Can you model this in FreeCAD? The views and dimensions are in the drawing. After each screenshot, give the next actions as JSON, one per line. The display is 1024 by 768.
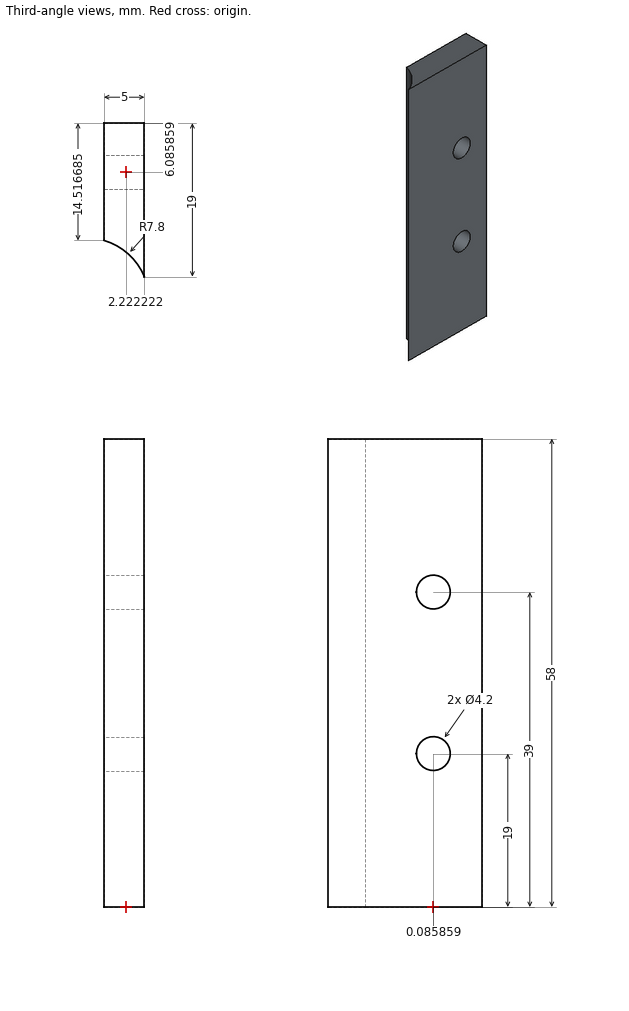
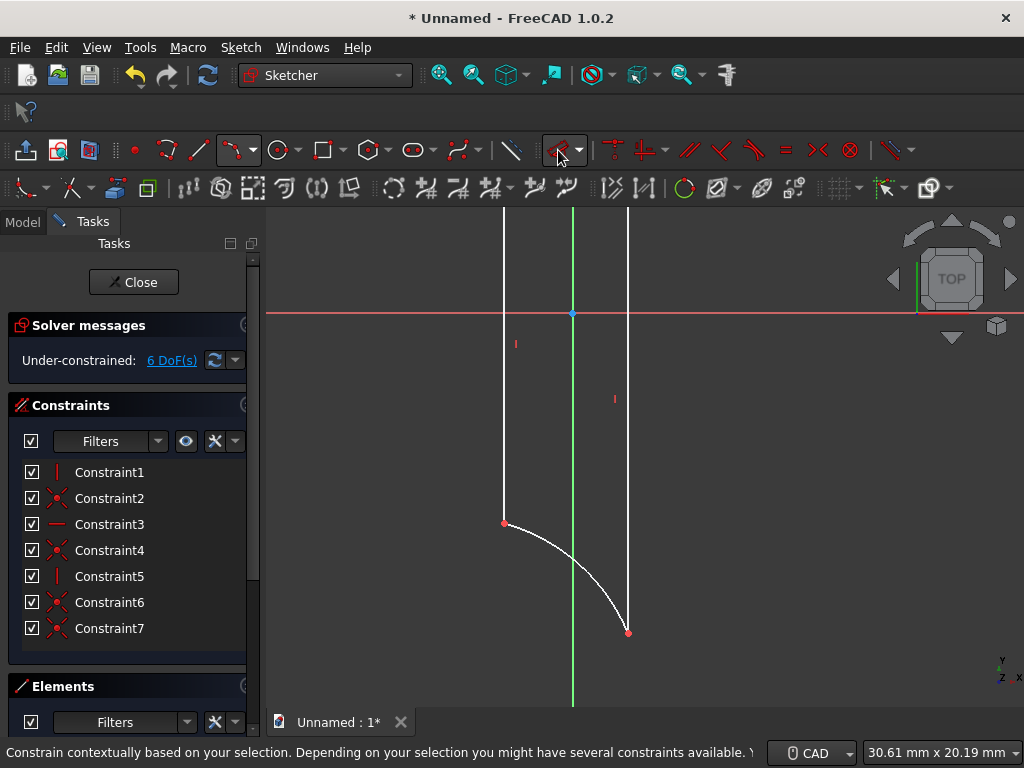
{"action": "left_click", "coordinate": [602, 589]}
{"action": "left_click", "coordinate": [671, 669]}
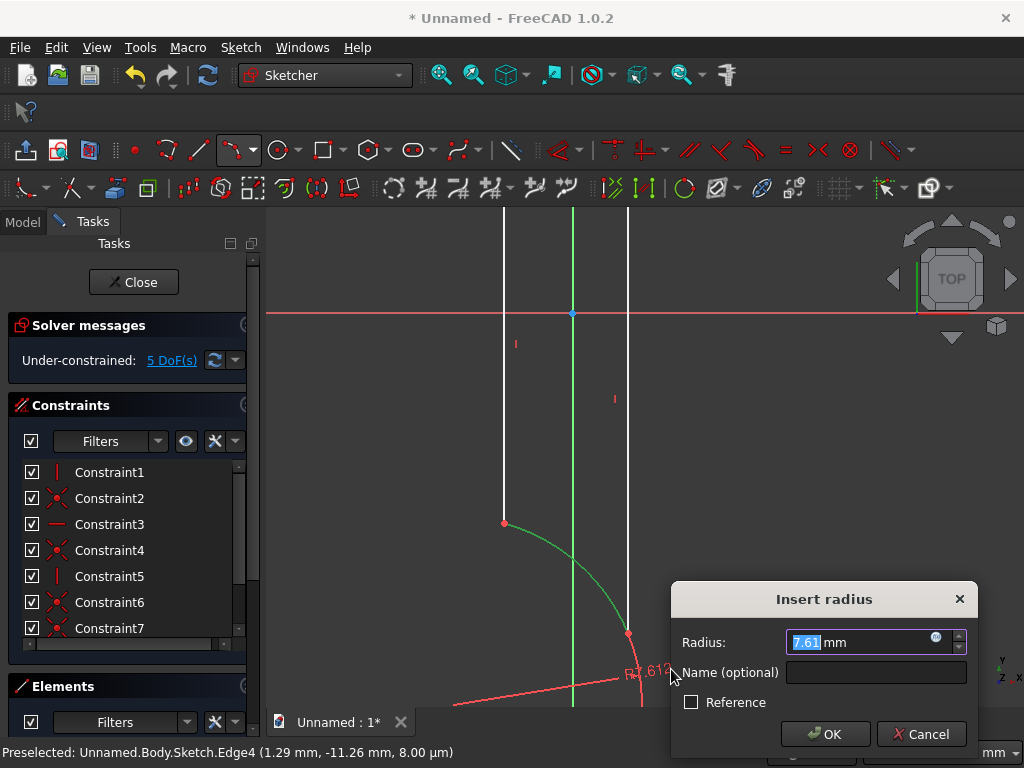
{"action": "type", "text": "7.8"}
{"action": "key", "text": "Return"}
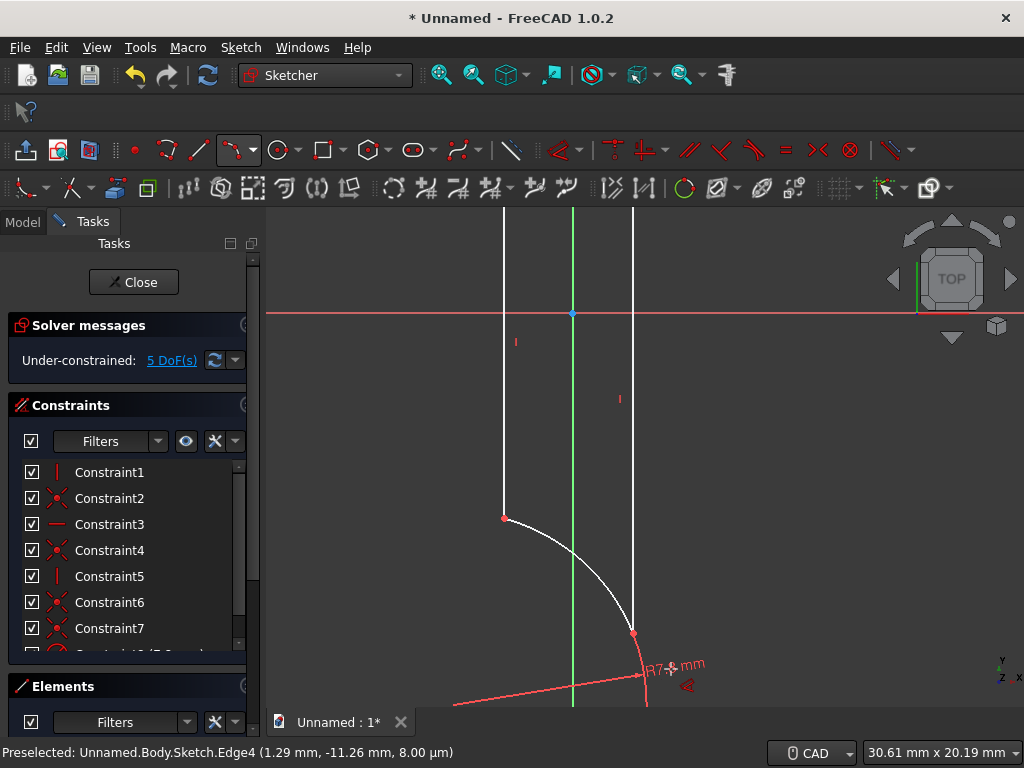
{"action": "scroll", "coordinate": [598, 578], "scroll_direction": "down", "scroll_amount": 2}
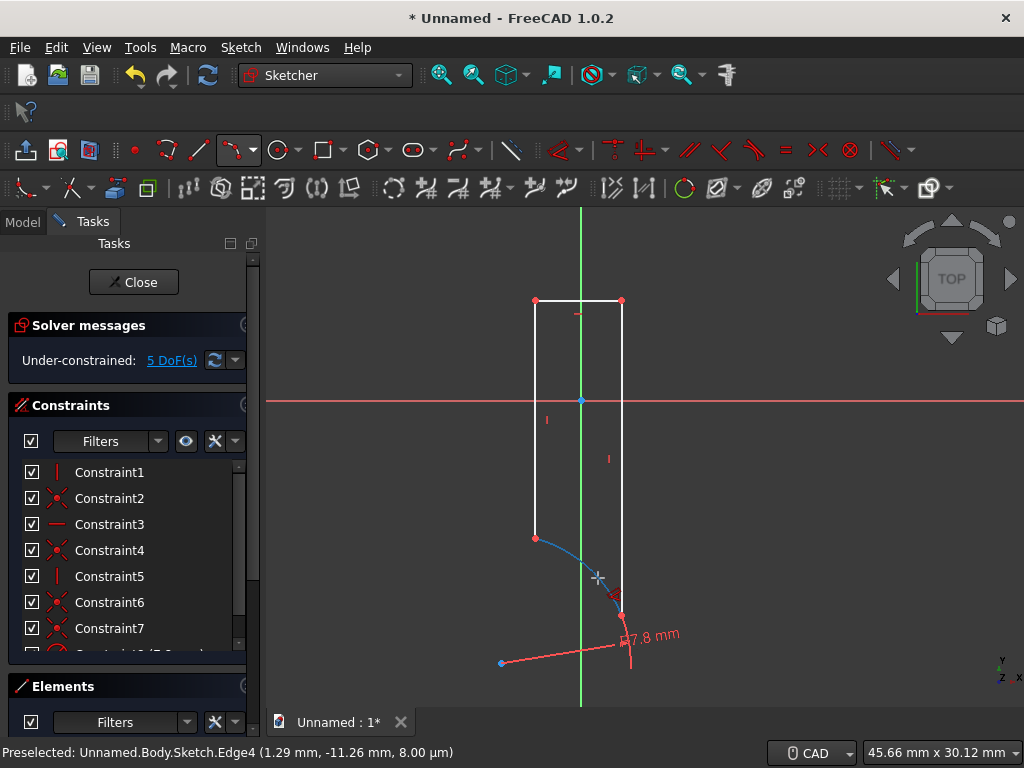
{"action": "left_click", "coordinate": [596, 301]}
{"action": "left_click", "coordinate": [559, 267]}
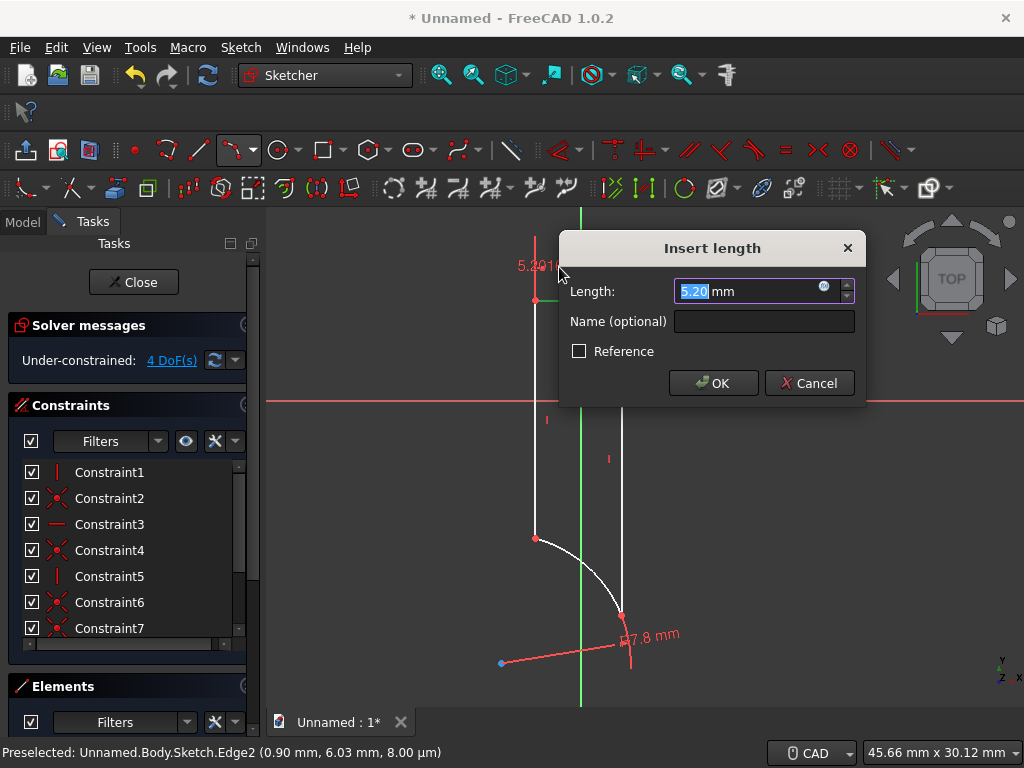
{"action": "type", "text": "5"}
{"action": "key", "text": "Return"}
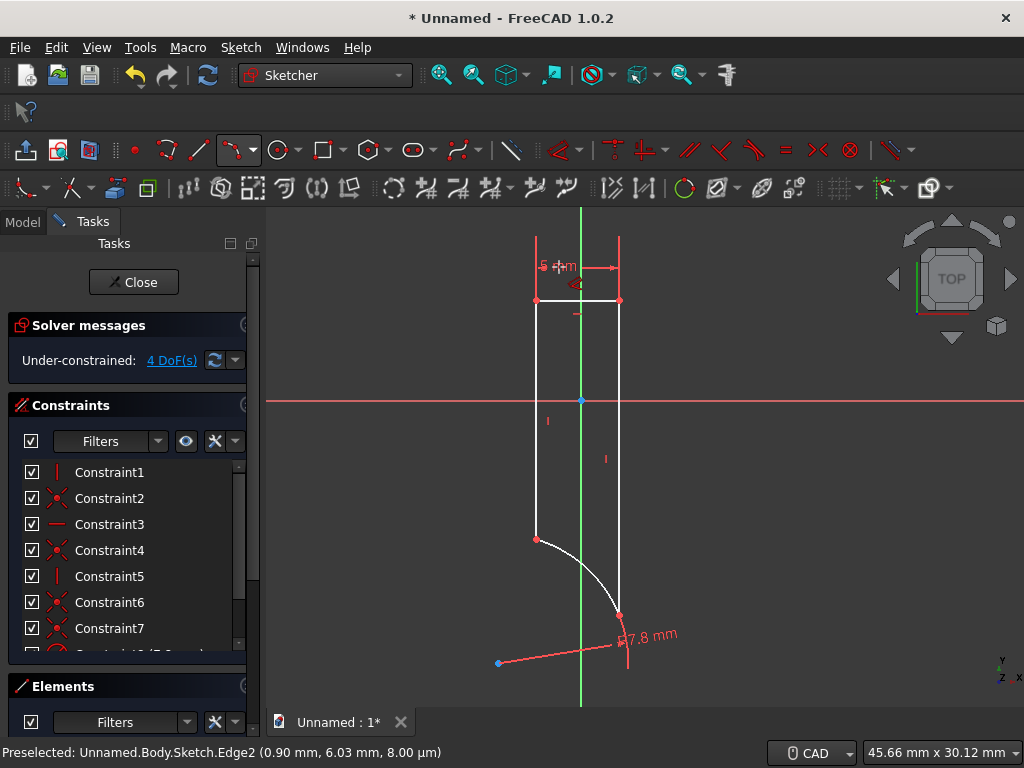
{"action": "left_click", "coordinate": [619, 521]}
{"action": "left_click", "coordinate": [653, 458]}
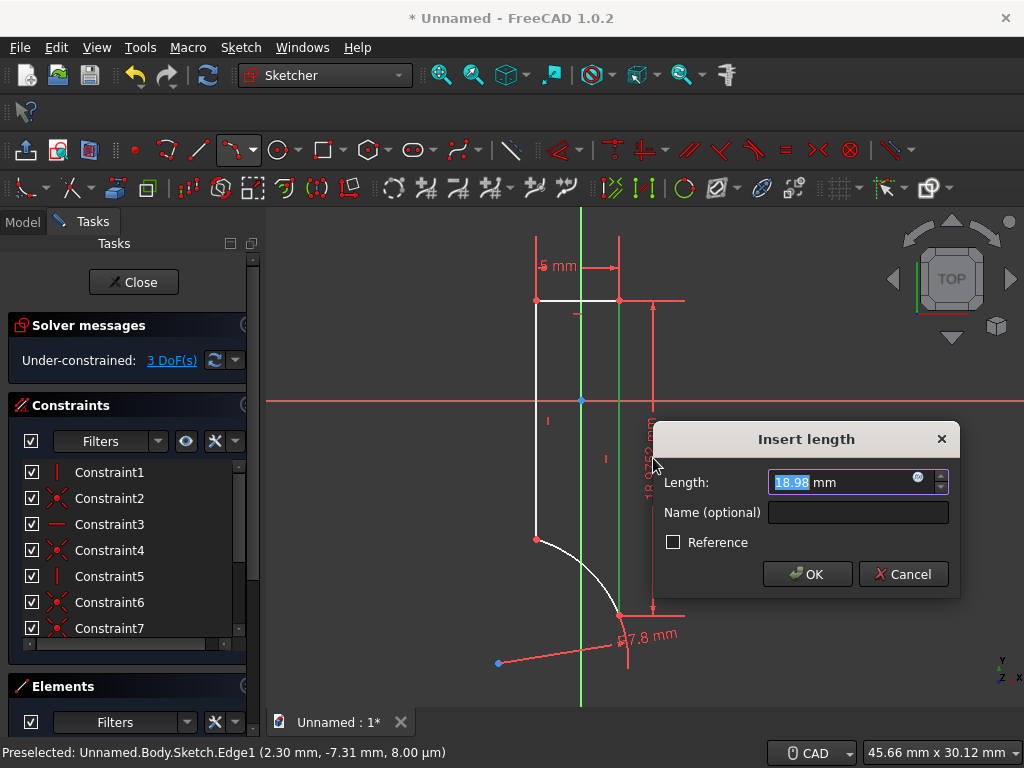
{"action": "type", "text": "19"}
{"action": "key", "text": "Return"}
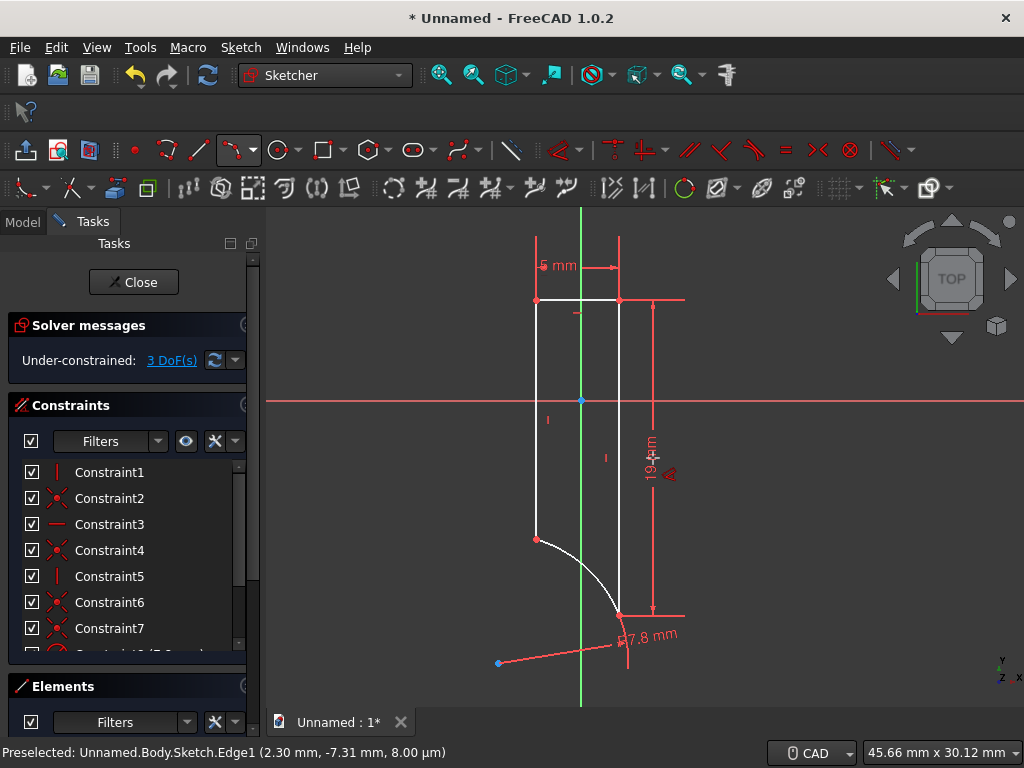
{"action": "left_click", "coordinate": [536, 372]}
{"action": "left_click", "coordinate": [502, 420]}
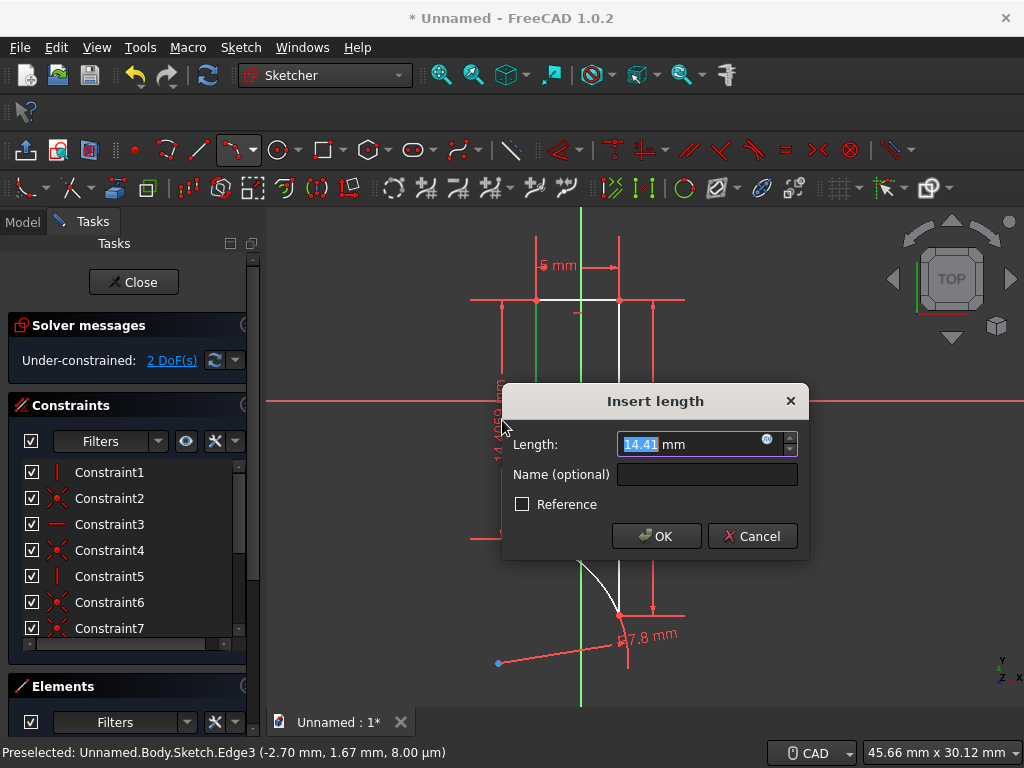
{"action": "type", "text": "14.516685"}
{"action": "key", "text": "Return"}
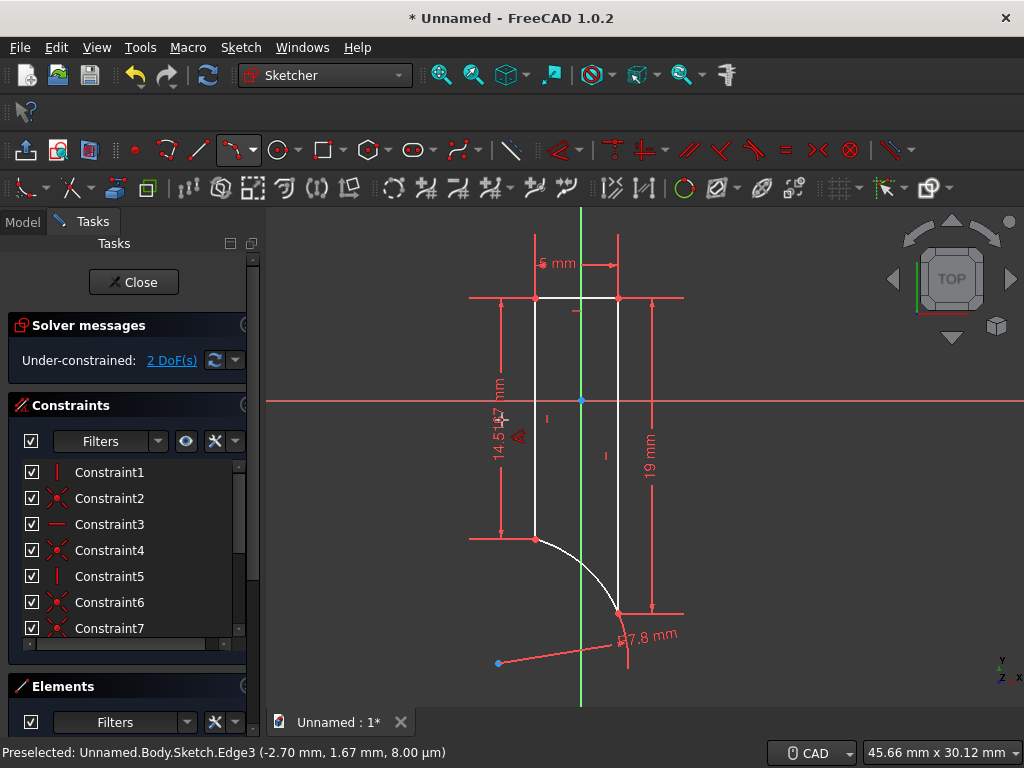
{"action": "left_click", "coordinate": [619, 614]}
{"action": "left_click", "coordinate": [600, 367]}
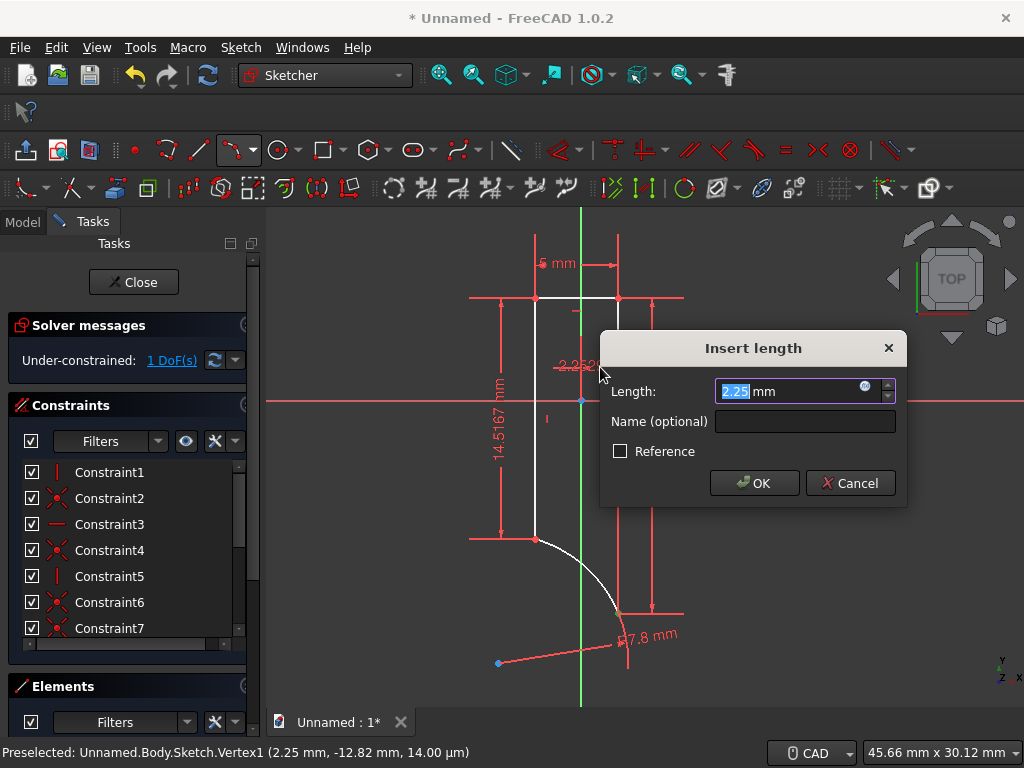
{"action": "type", "text": "2.222222"}
{"action": "key", "text": "Return"}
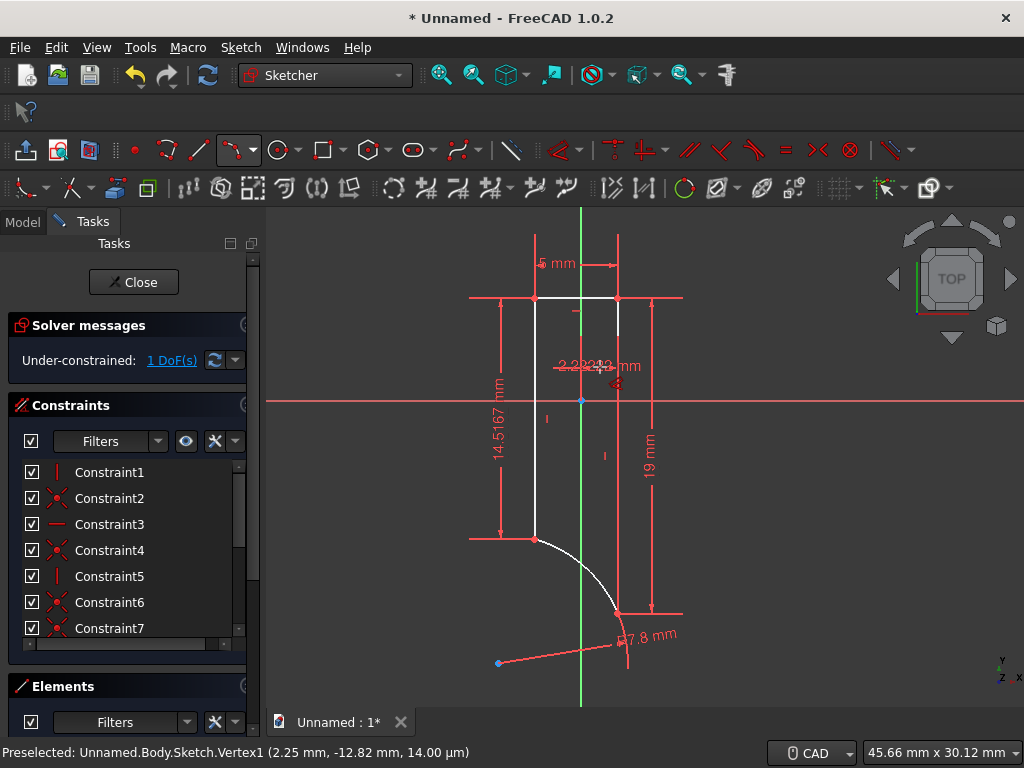
{"action": "left_click", "coordinate": [618, 298]}
{"action": "left_click", "coordinate": [652, 326]}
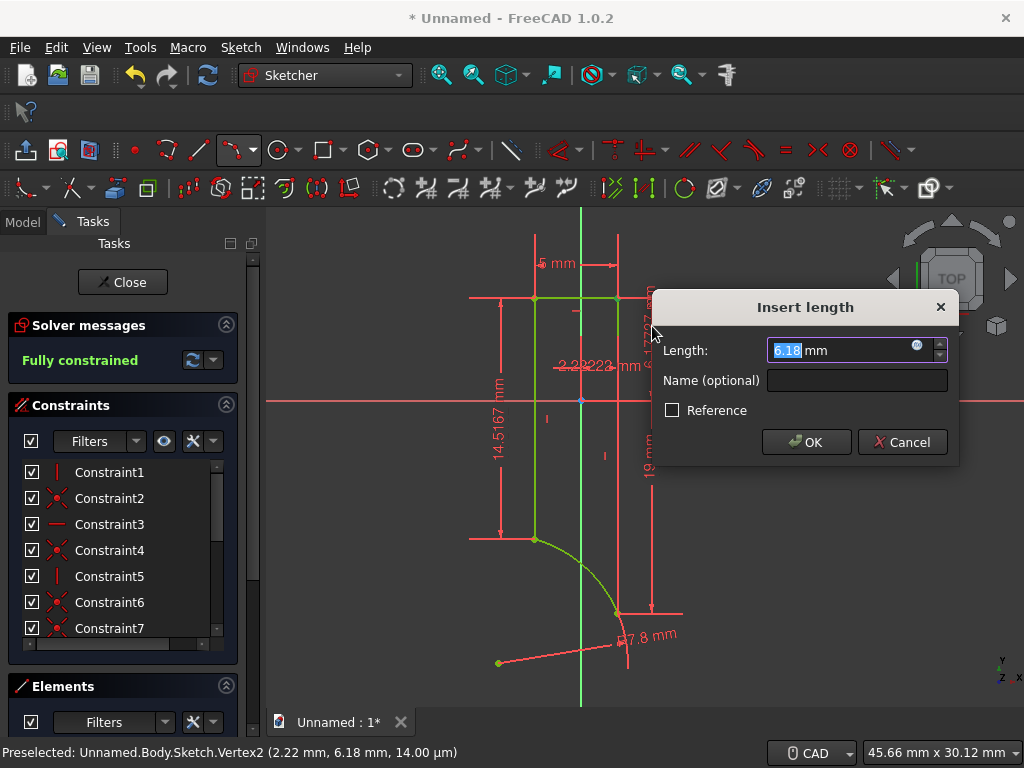
{"action": "type", "text": "6.085859"}
{"action": "key", "text": "Return"}
{"action": "key", "text": "Escape"}